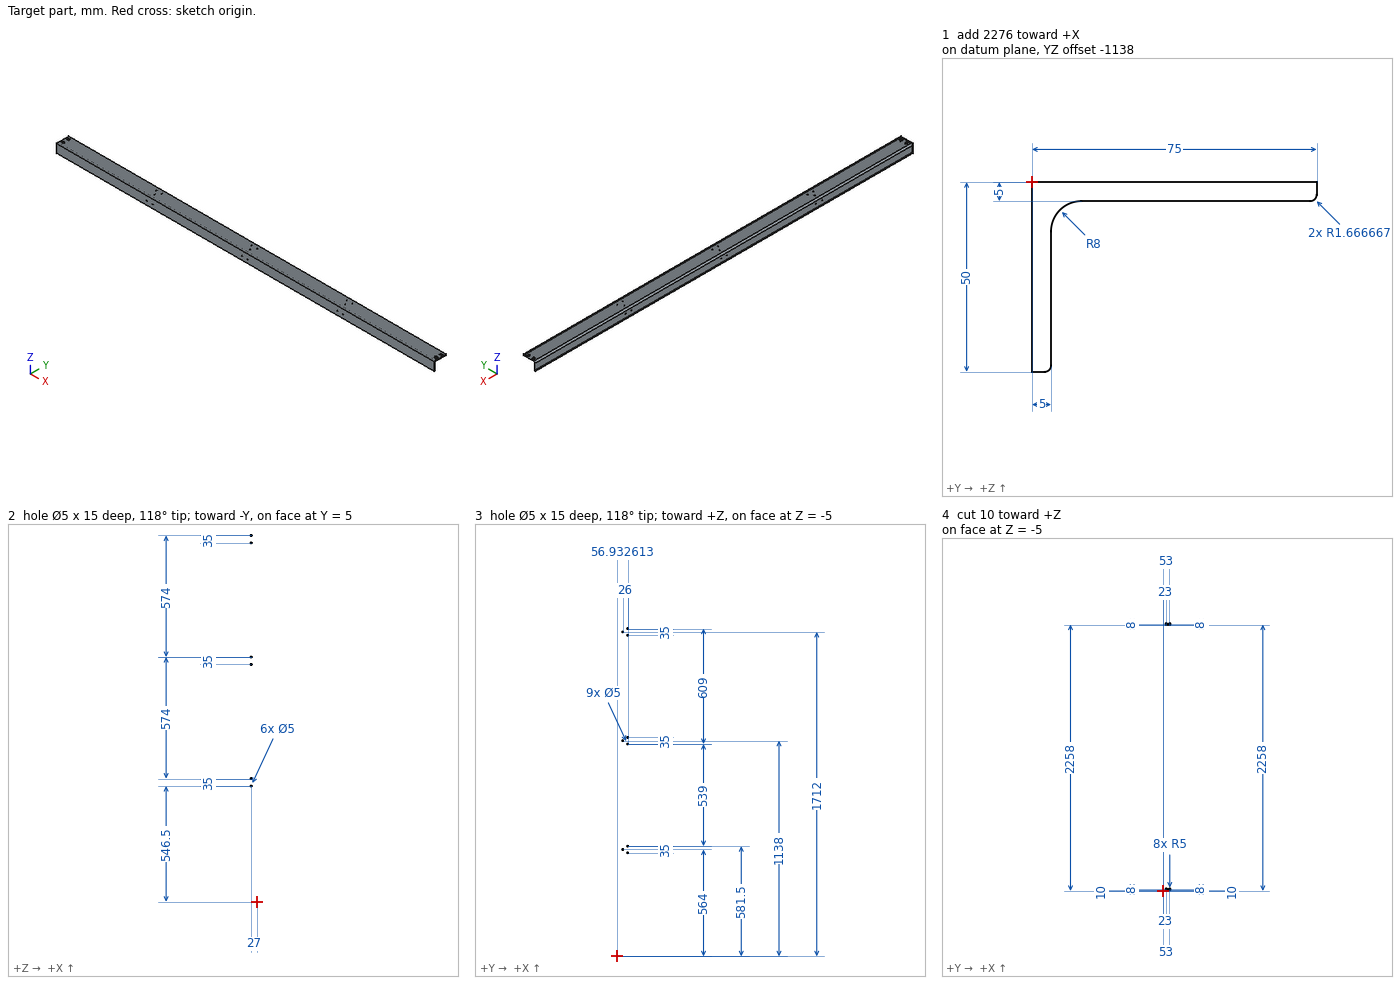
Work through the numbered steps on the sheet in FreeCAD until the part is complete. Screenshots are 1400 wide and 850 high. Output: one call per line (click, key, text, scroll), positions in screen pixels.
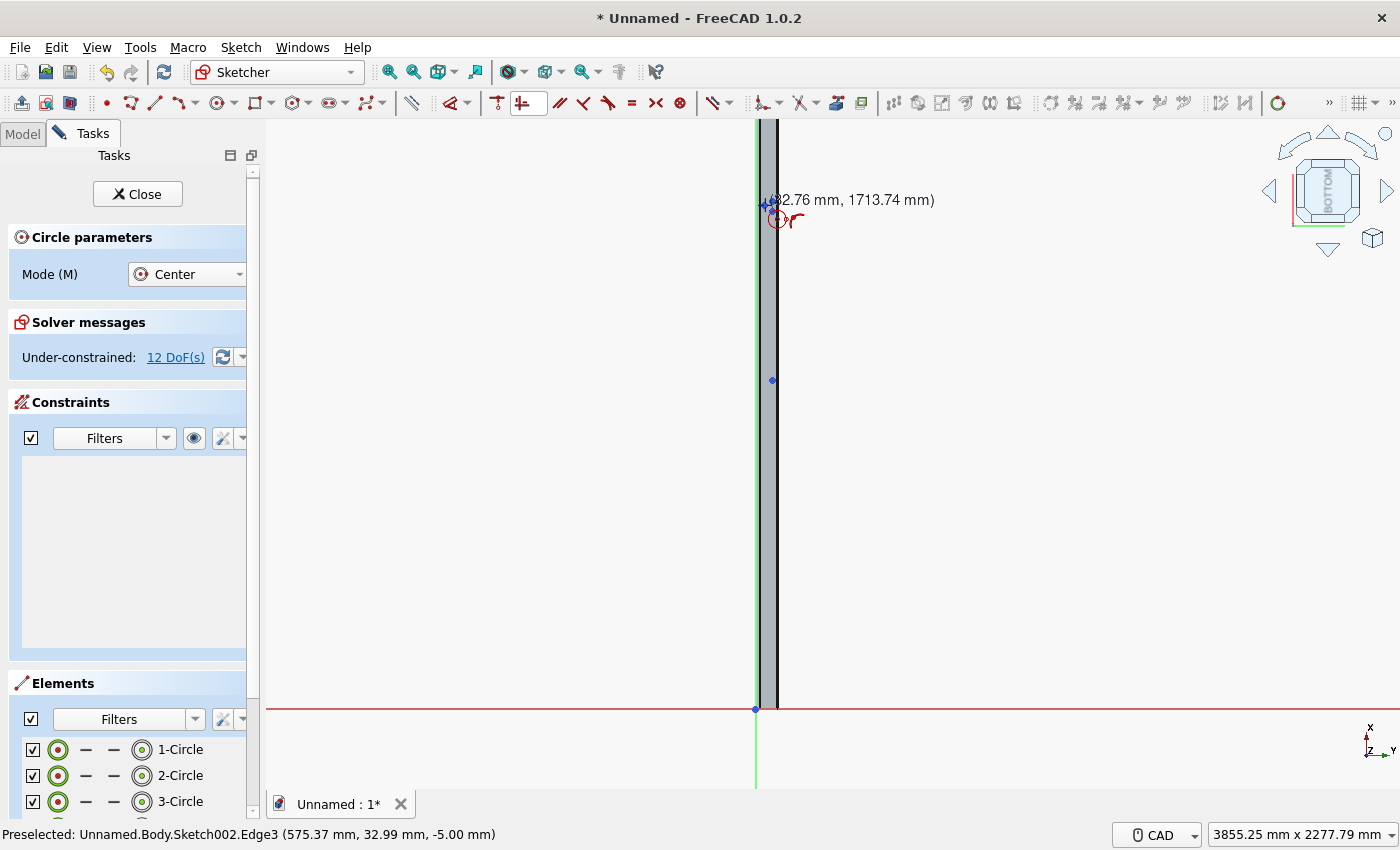
scroll(773, 538, up, 18)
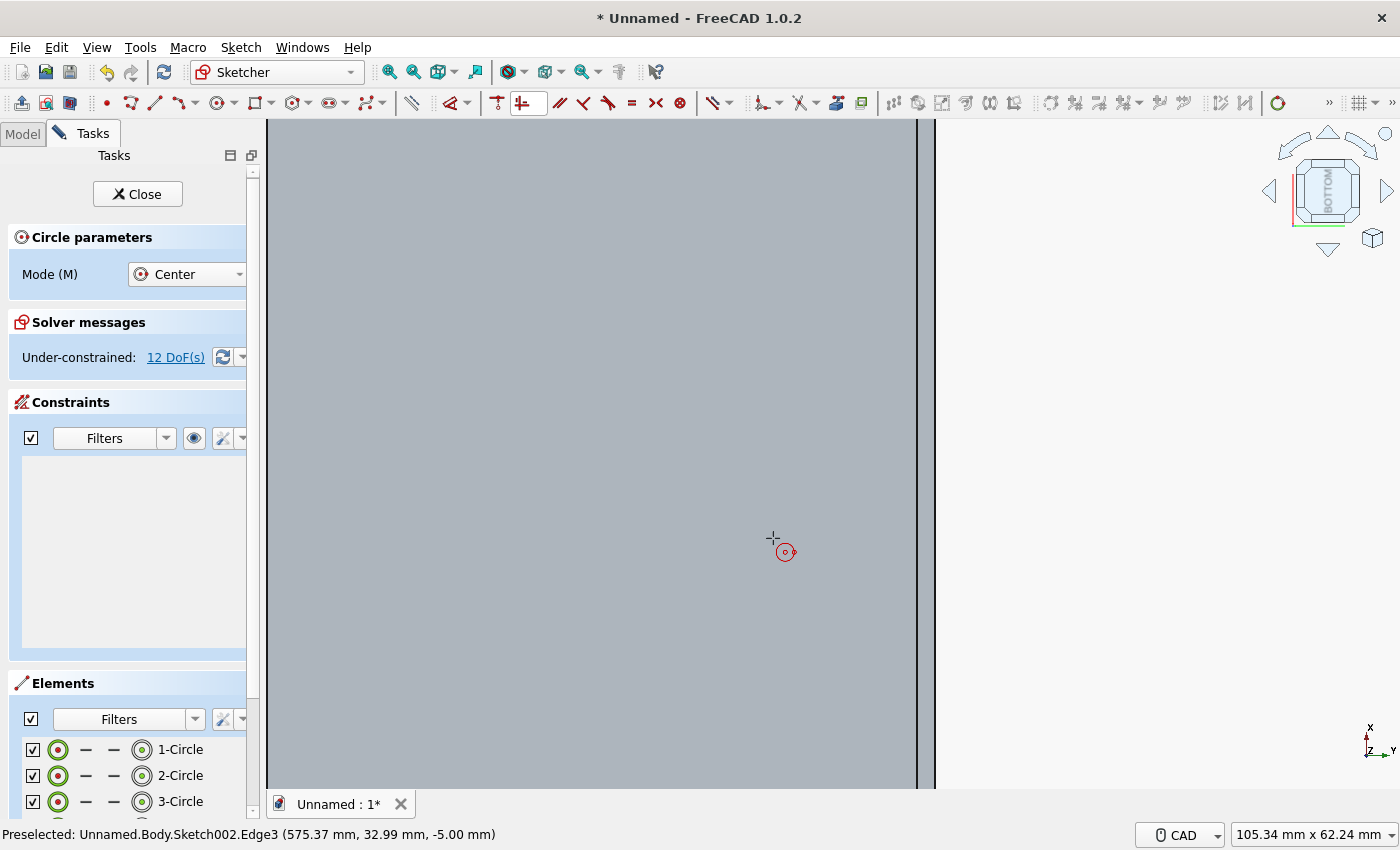
scroll(773, 538, down, 18)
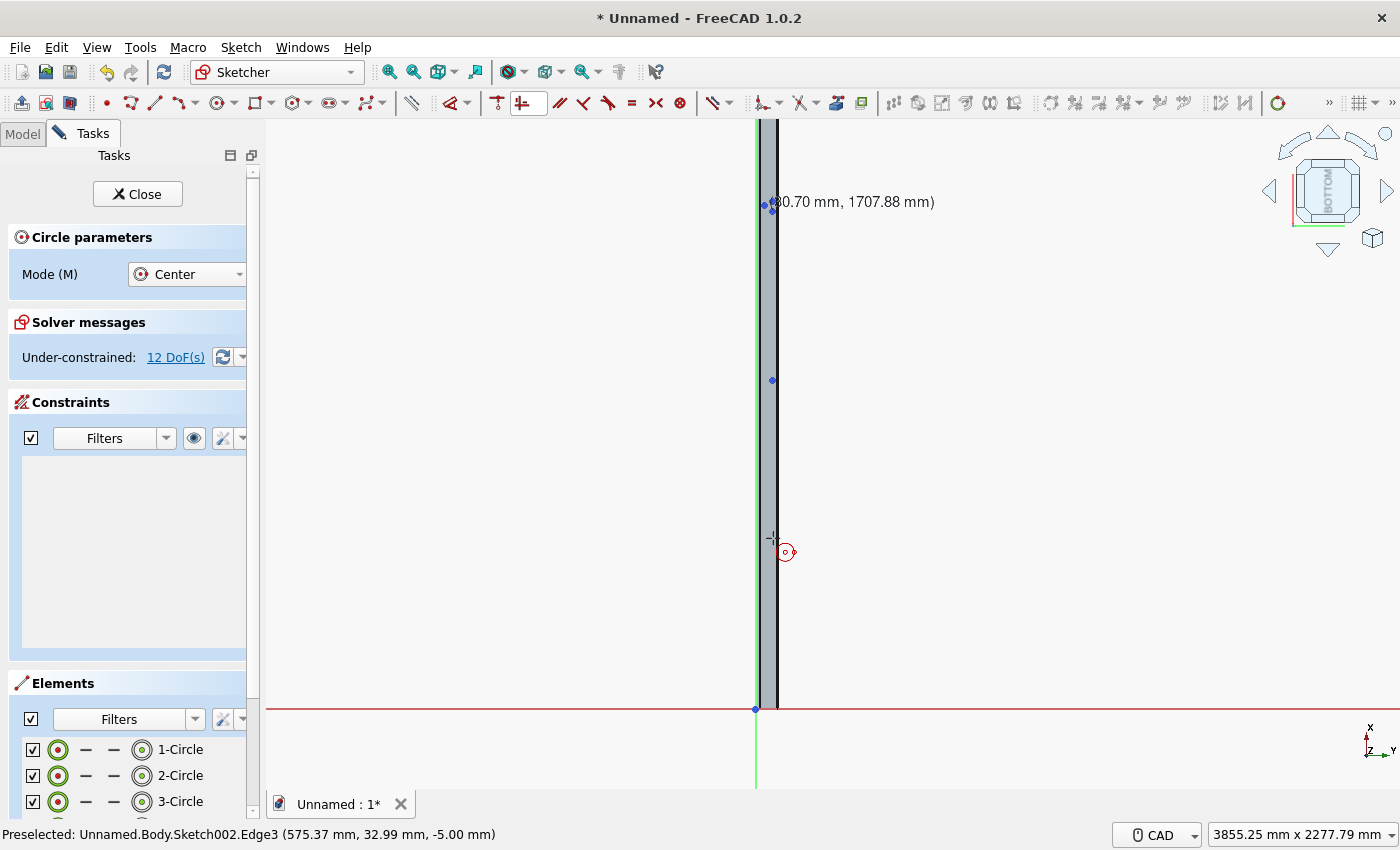
click(773, 538)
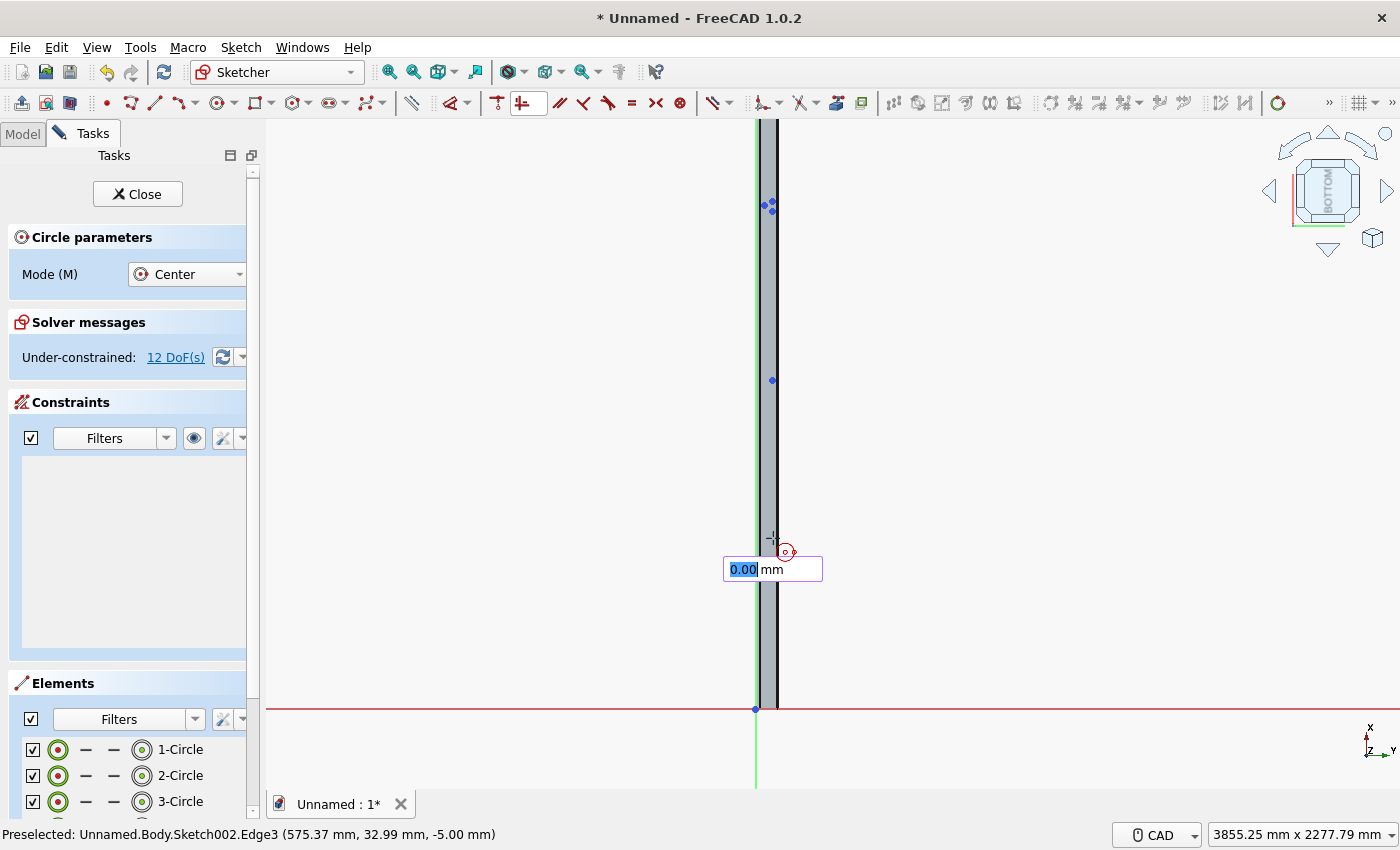
scroll(773, 538, up, 16)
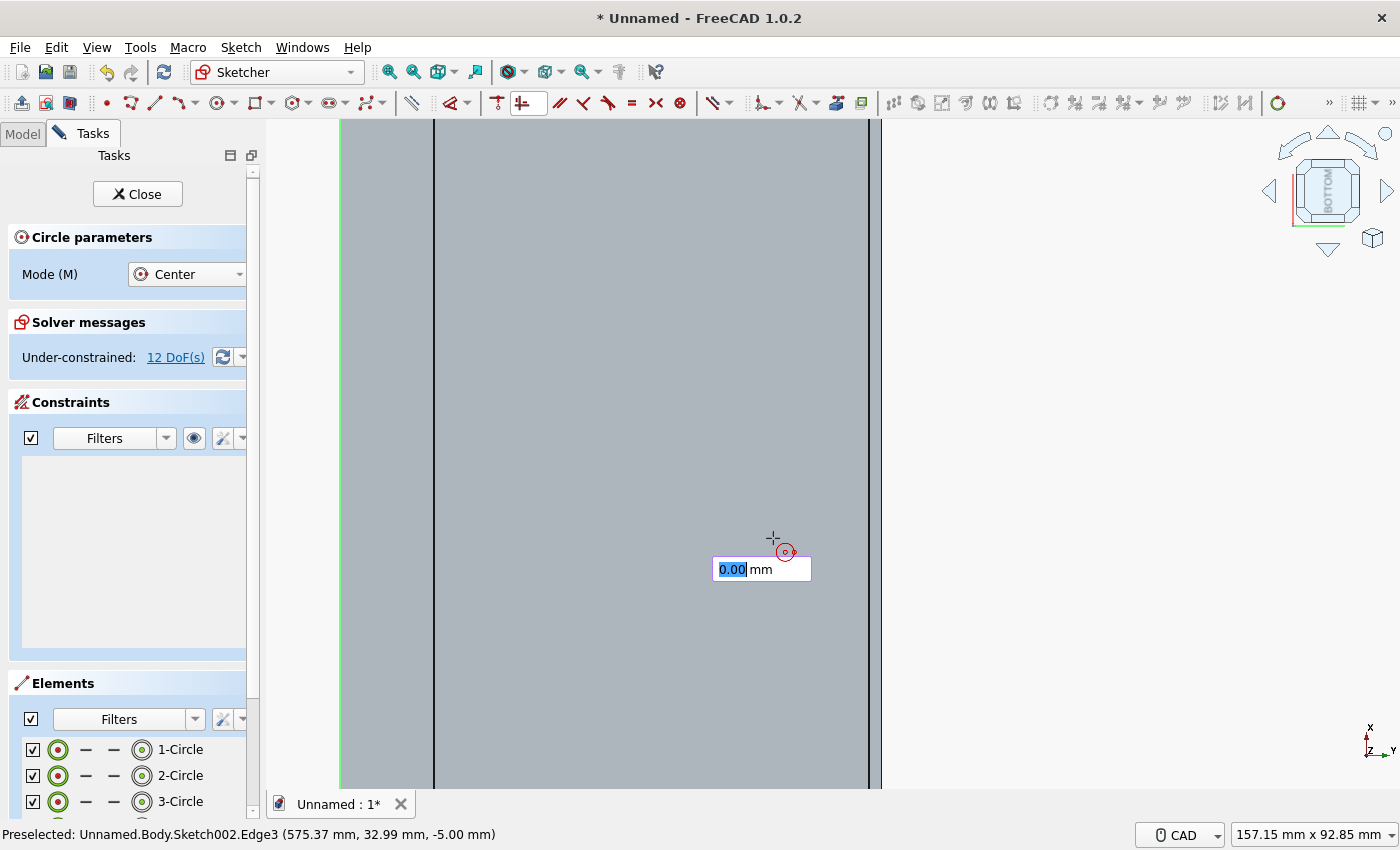
click(764, 516)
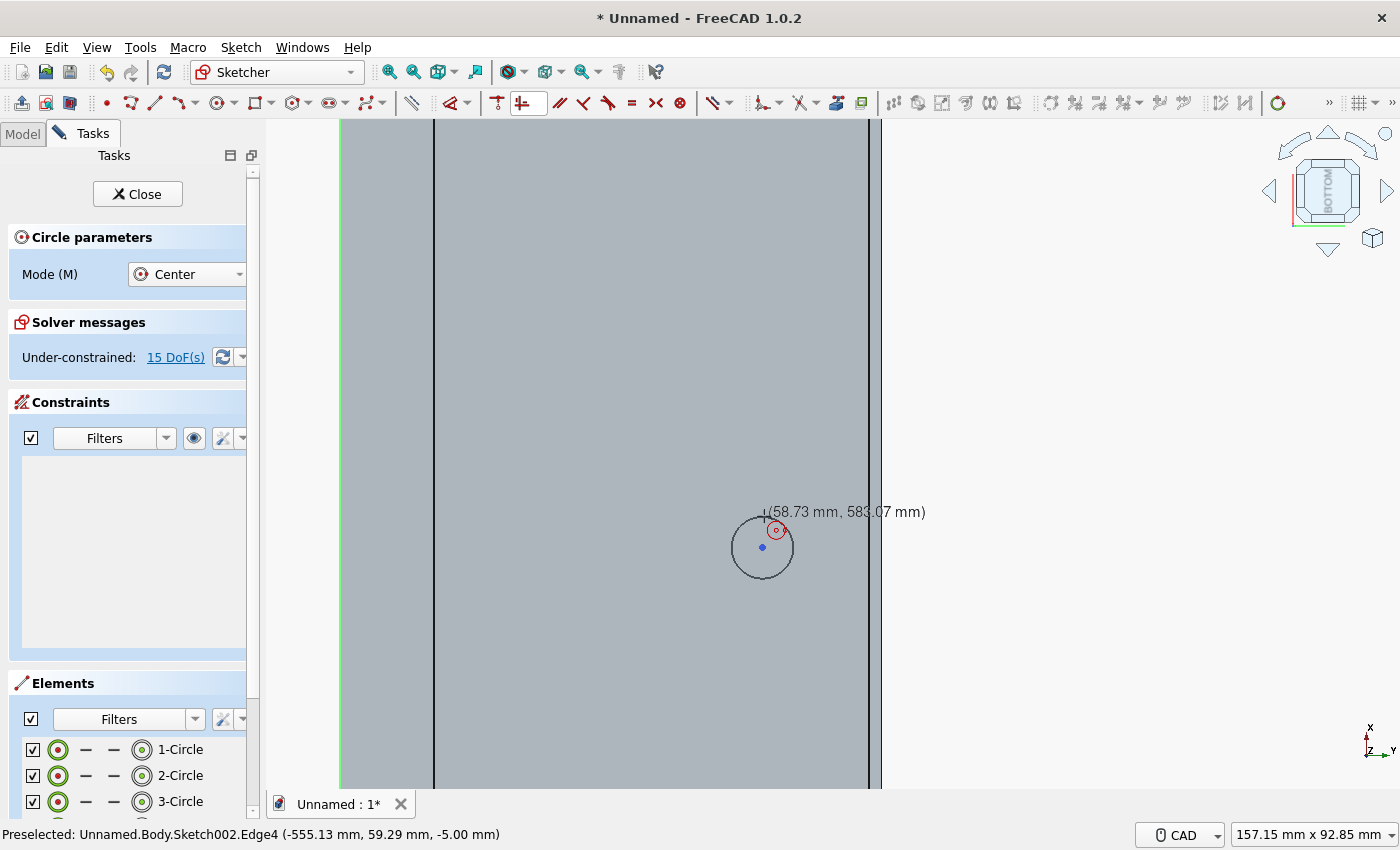
scroll(773, 538, down, 16)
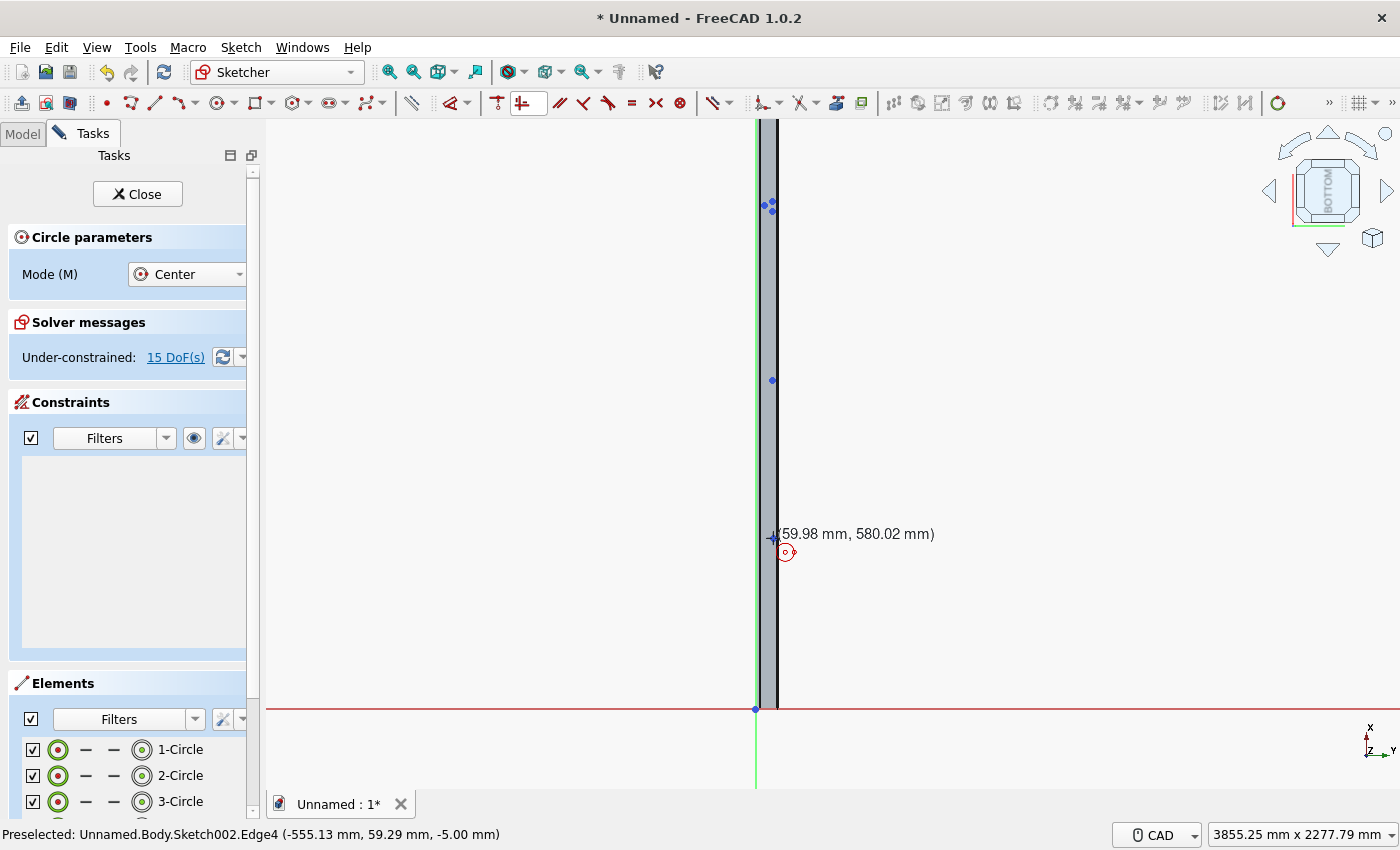
scroll(773, 549, up, 18)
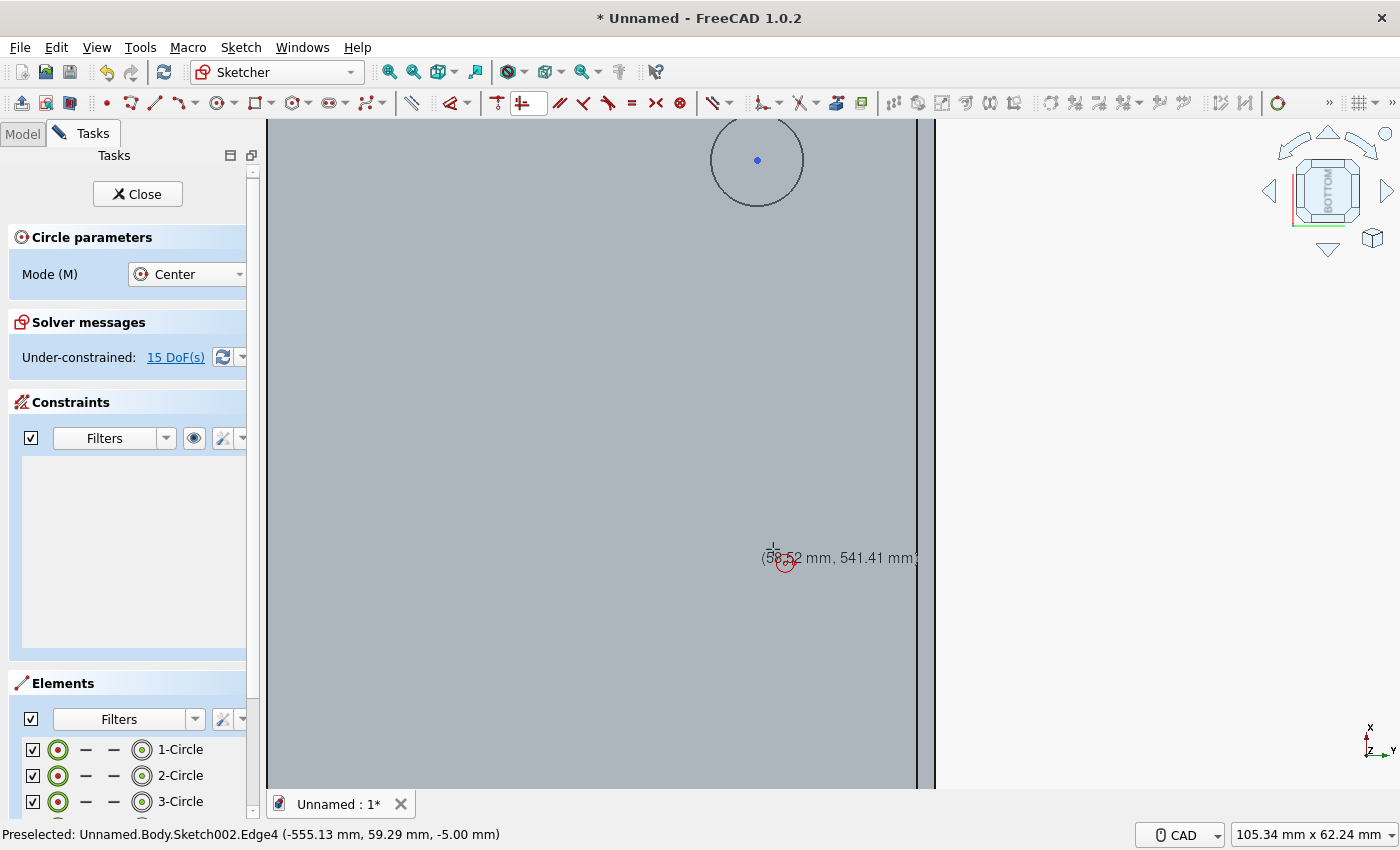
scroll(773, 549, down, 18)